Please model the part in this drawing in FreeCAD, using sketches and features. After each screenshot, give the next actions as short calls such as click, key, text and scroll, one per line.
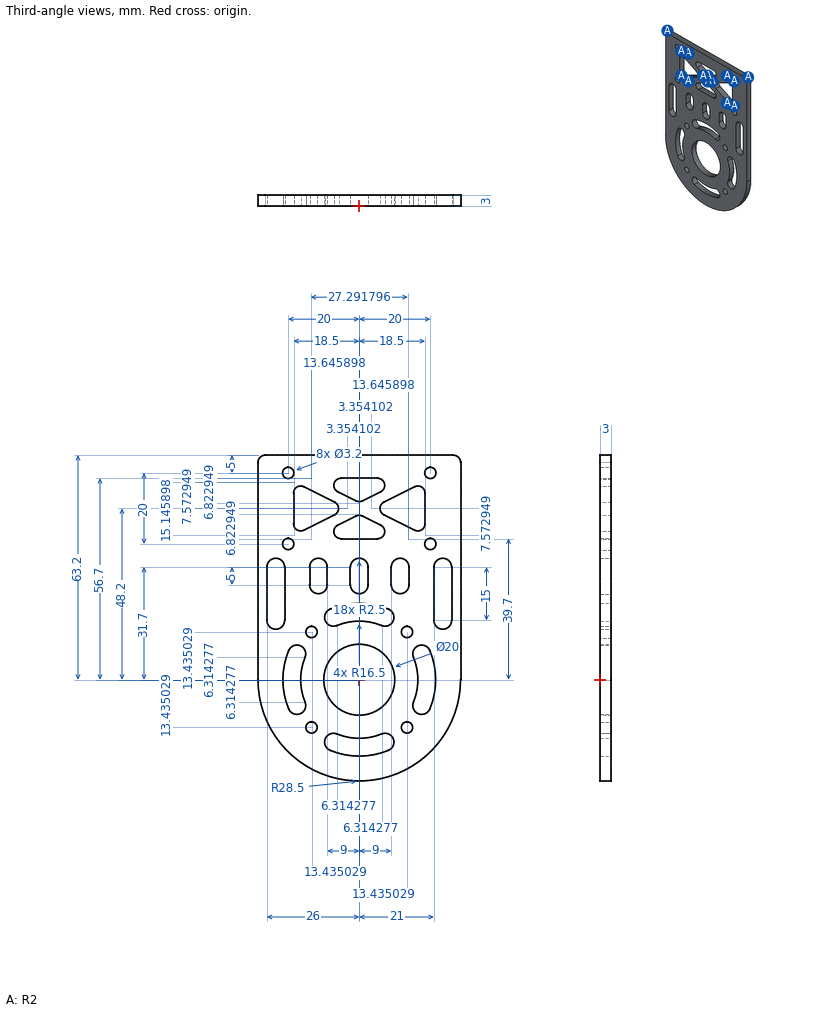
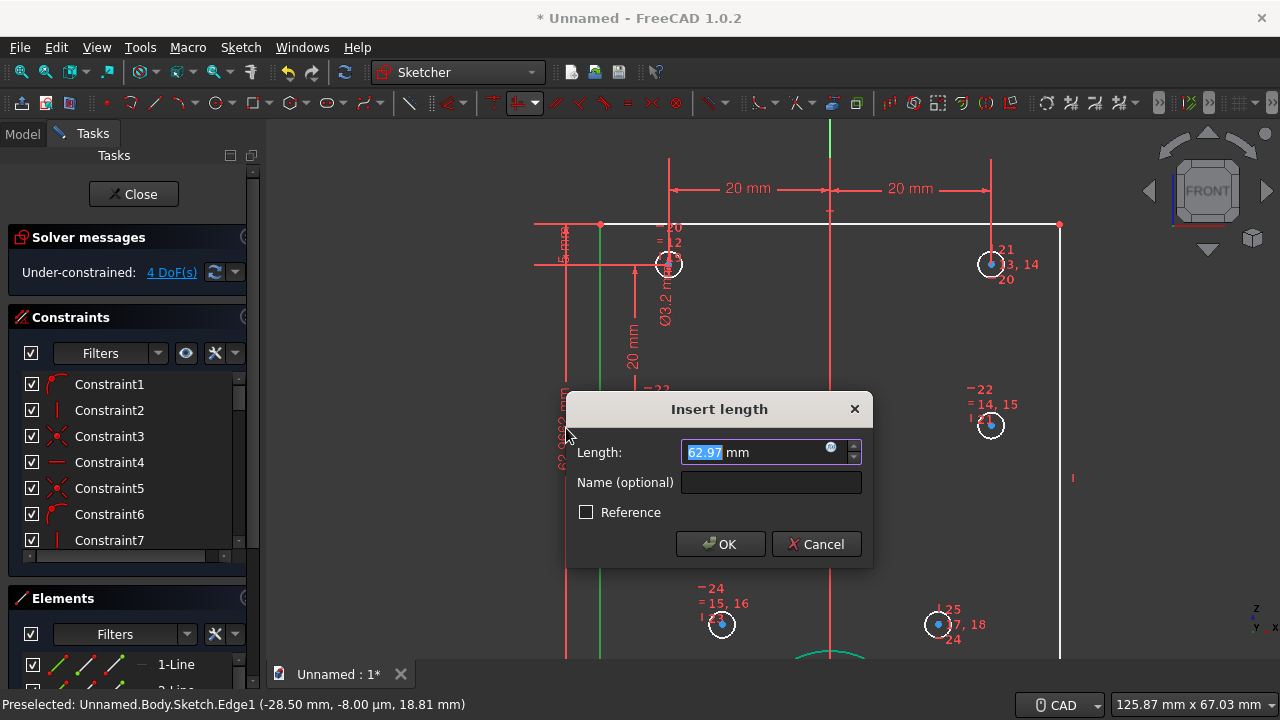
text(63.2)
key(Return)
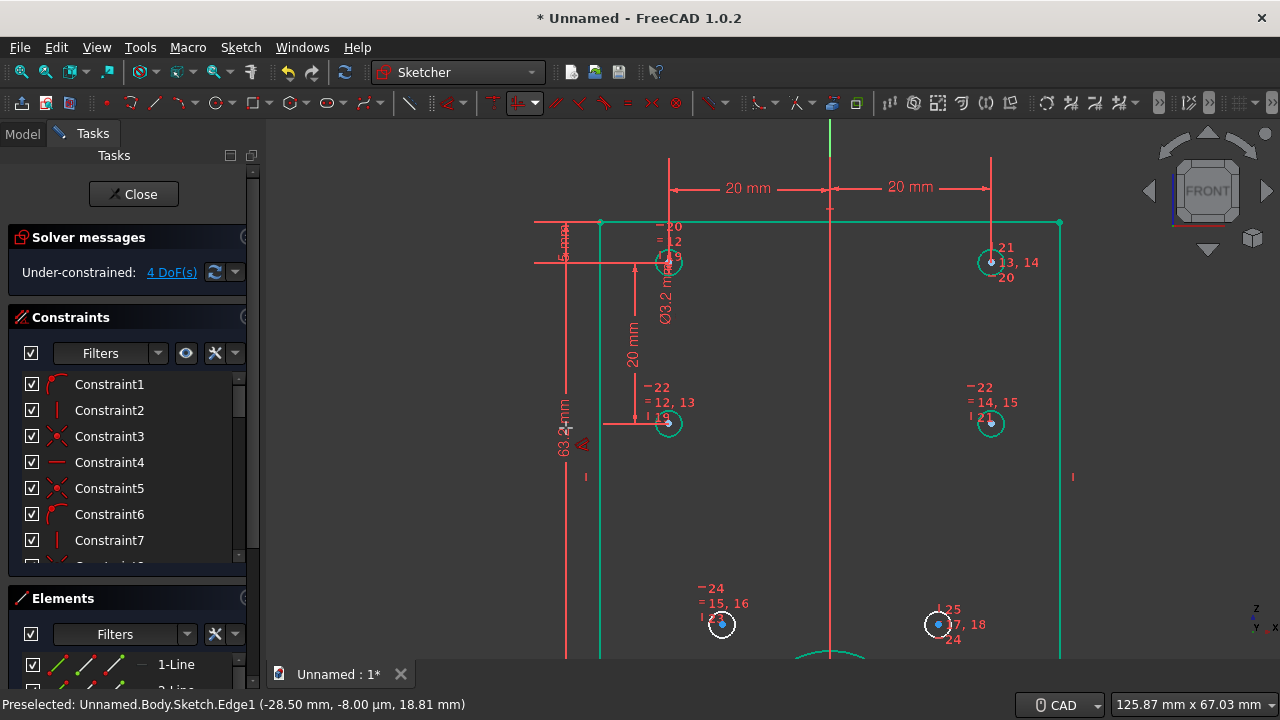
click(722, 625)
click(776, 591)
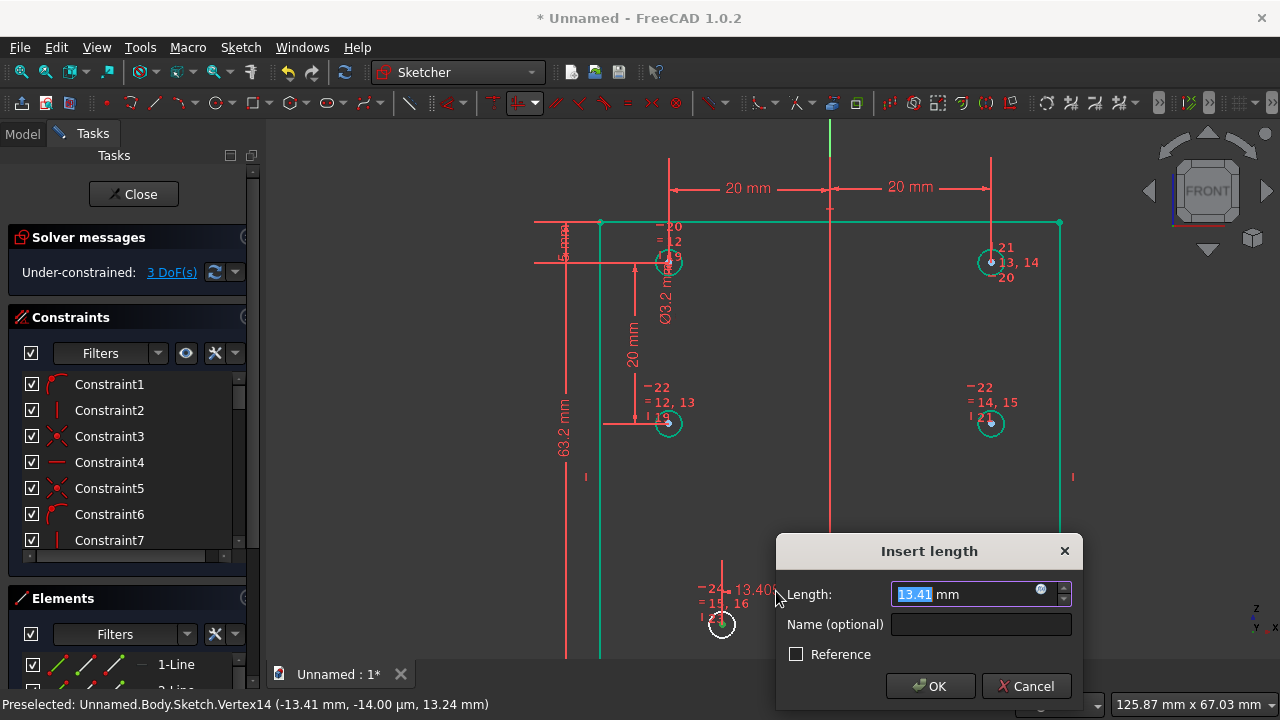
text(13.435029)
key(Return)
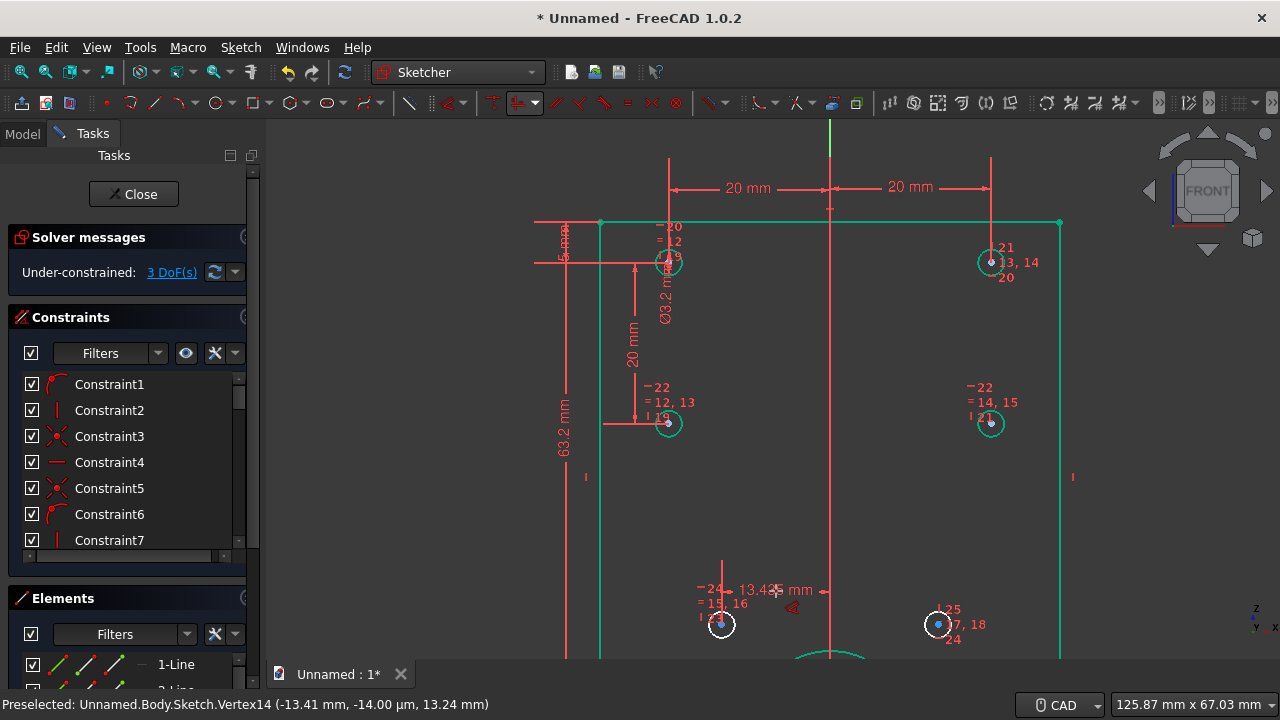
click(722, 625)
click(688, 628)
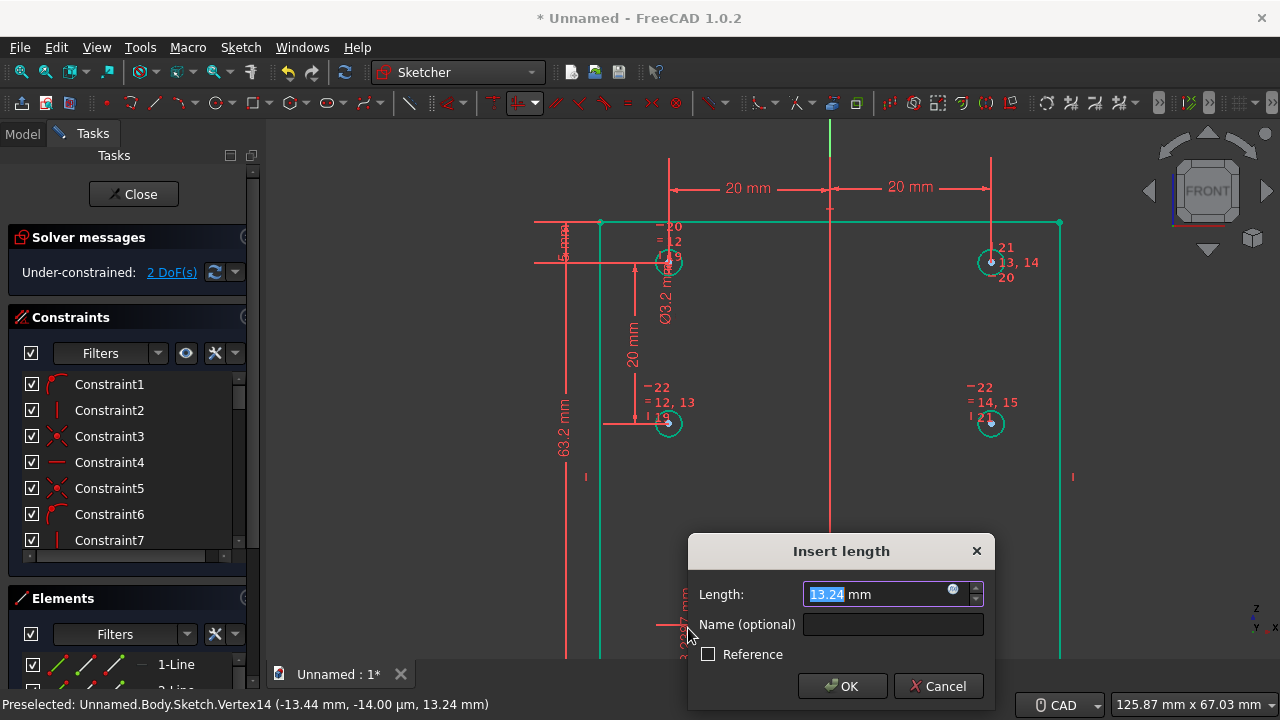
text(13.435029)
key(Return)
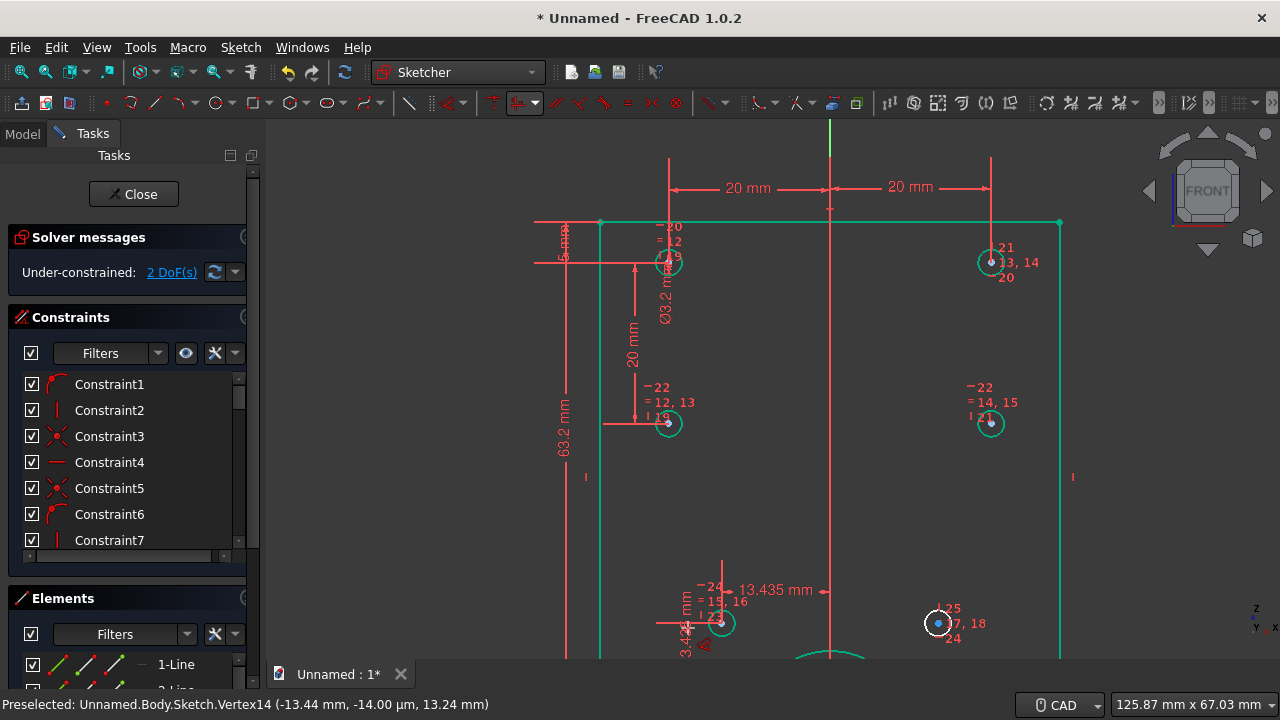
scroll(602, 224, down, 4)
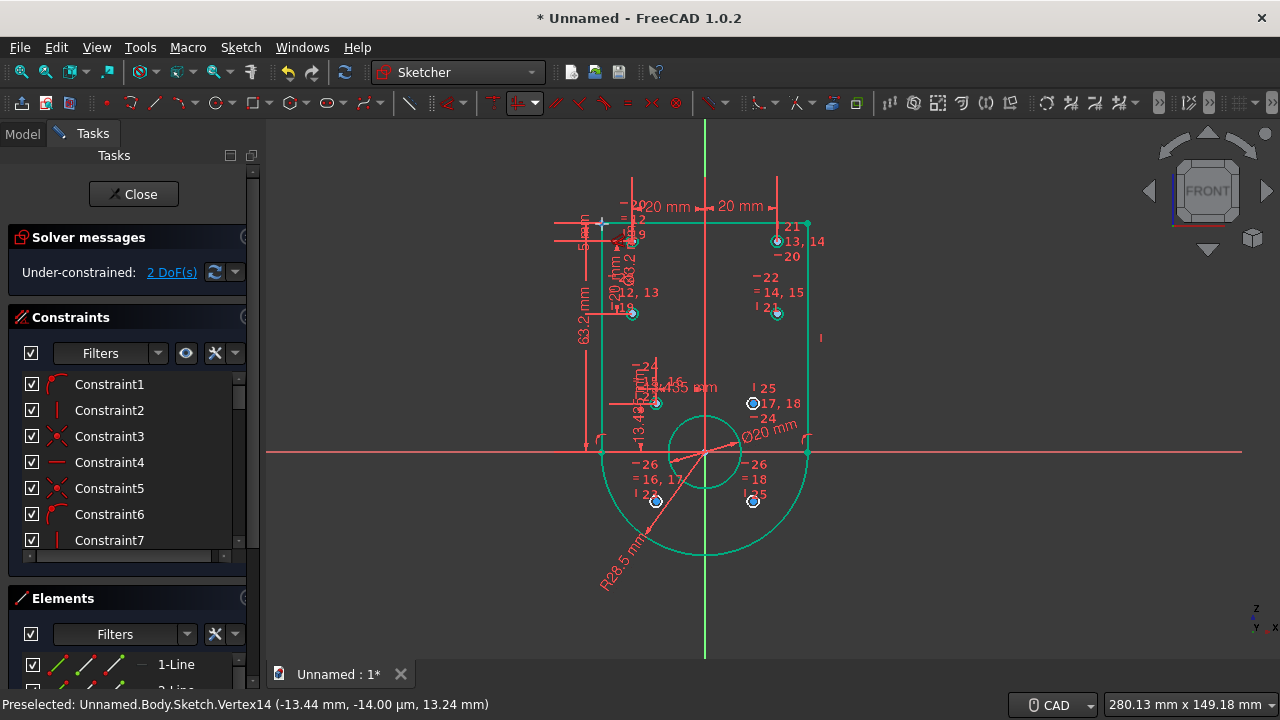
click(656, 501)
click(622, 477)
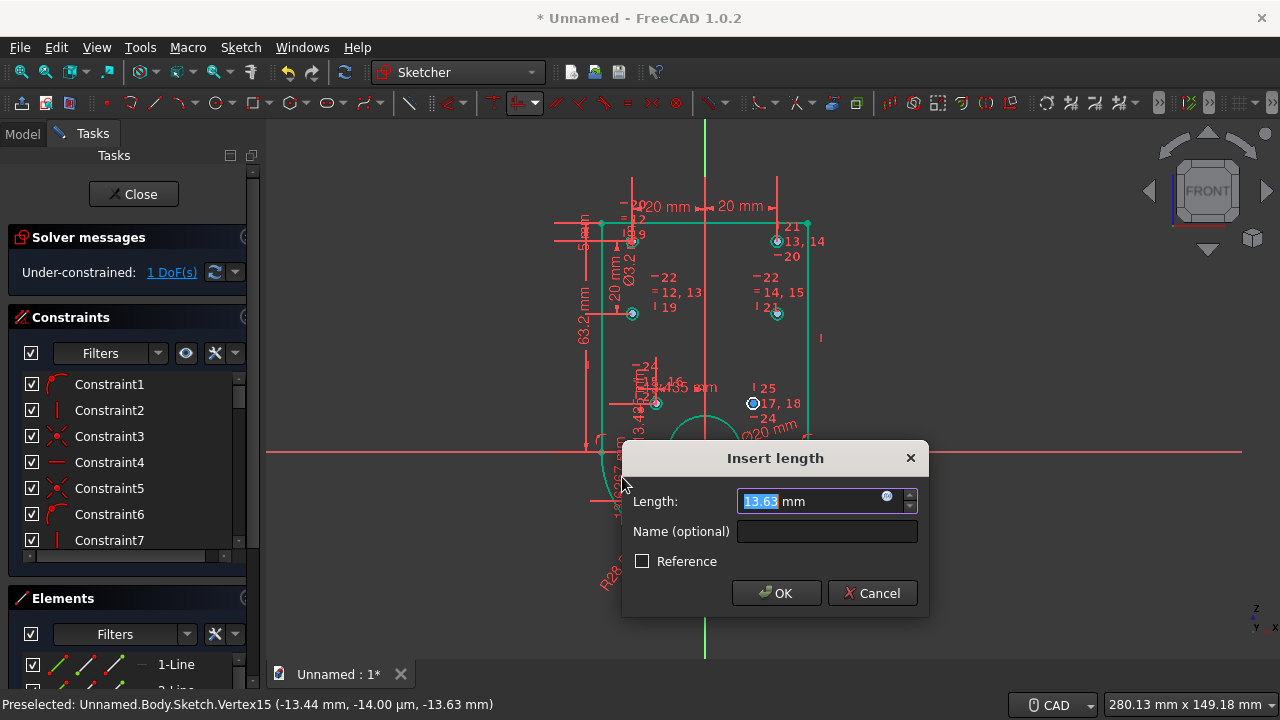
text(13.435029)
key(Return)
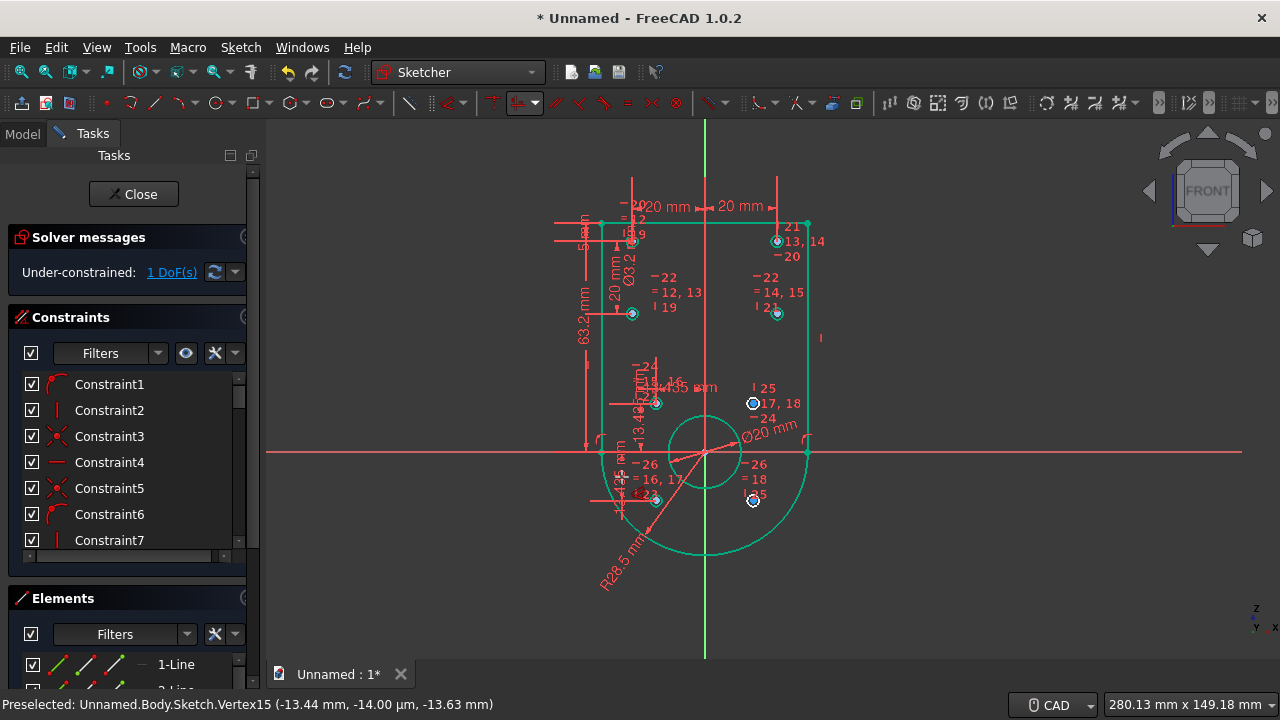
click(753, 404)
click(729, 510)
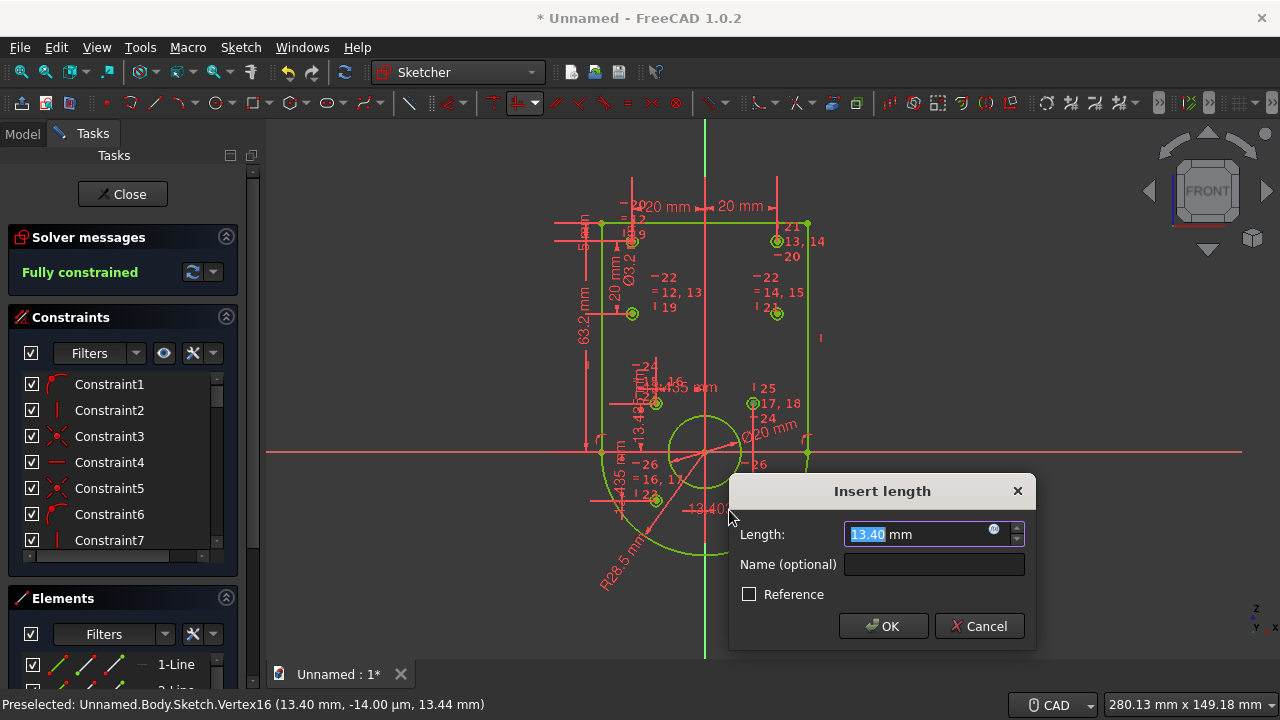
text(13.435029)
key(Return)
key(Escape)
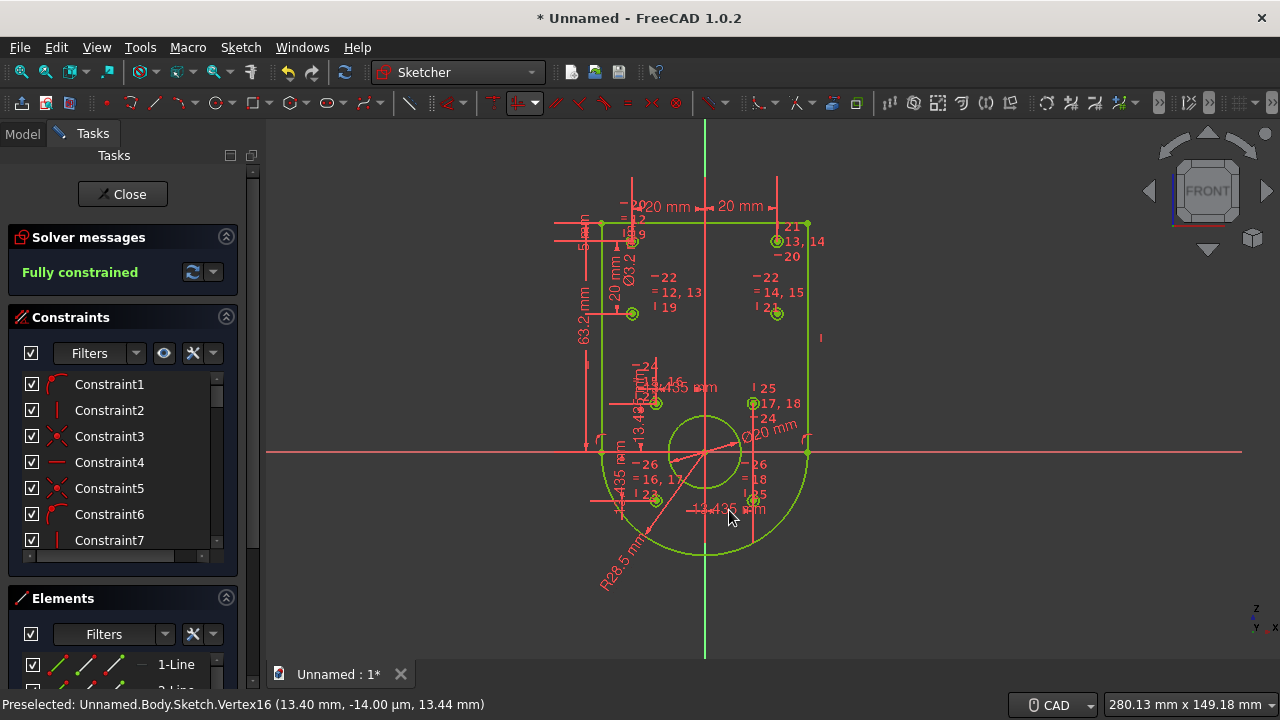
click(123, 194)